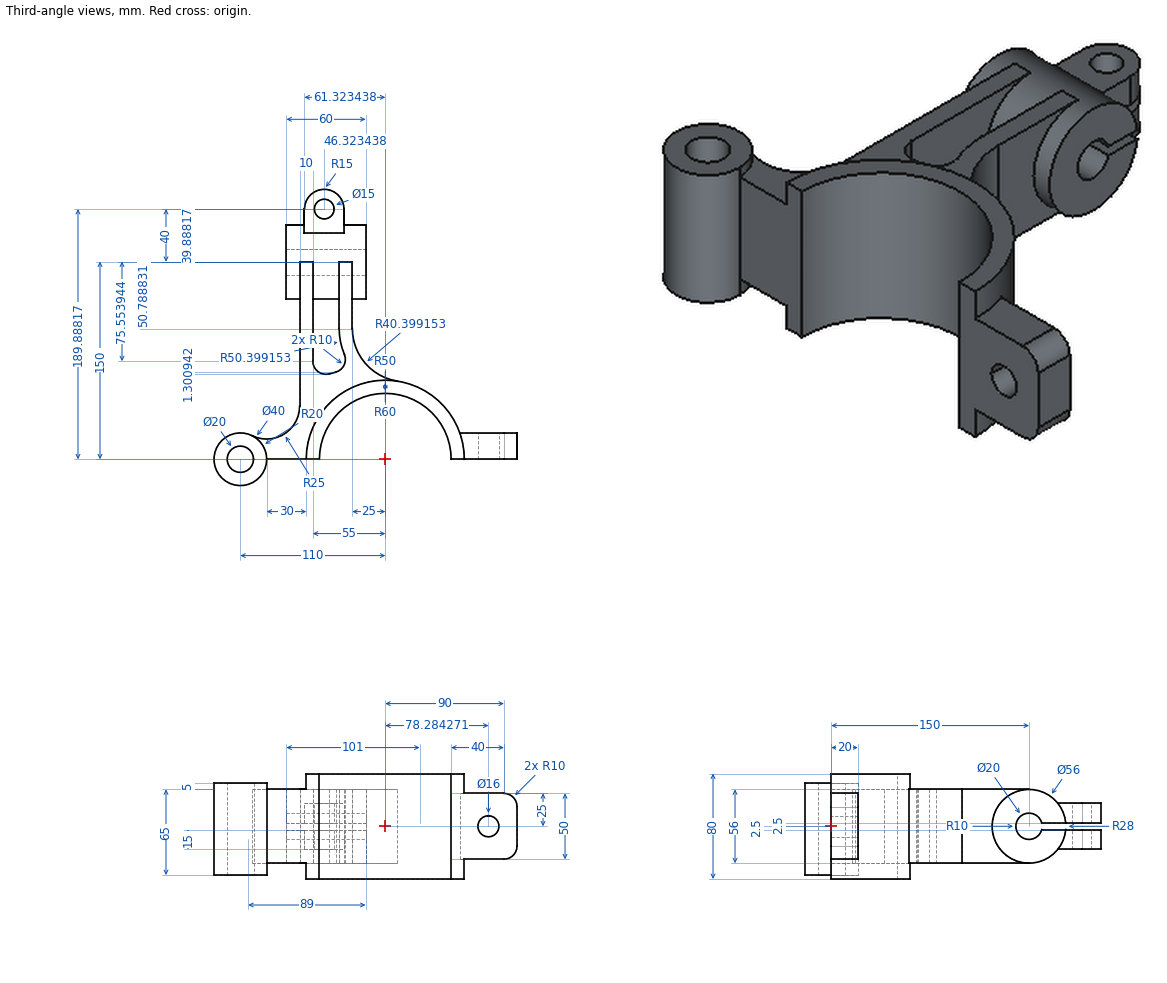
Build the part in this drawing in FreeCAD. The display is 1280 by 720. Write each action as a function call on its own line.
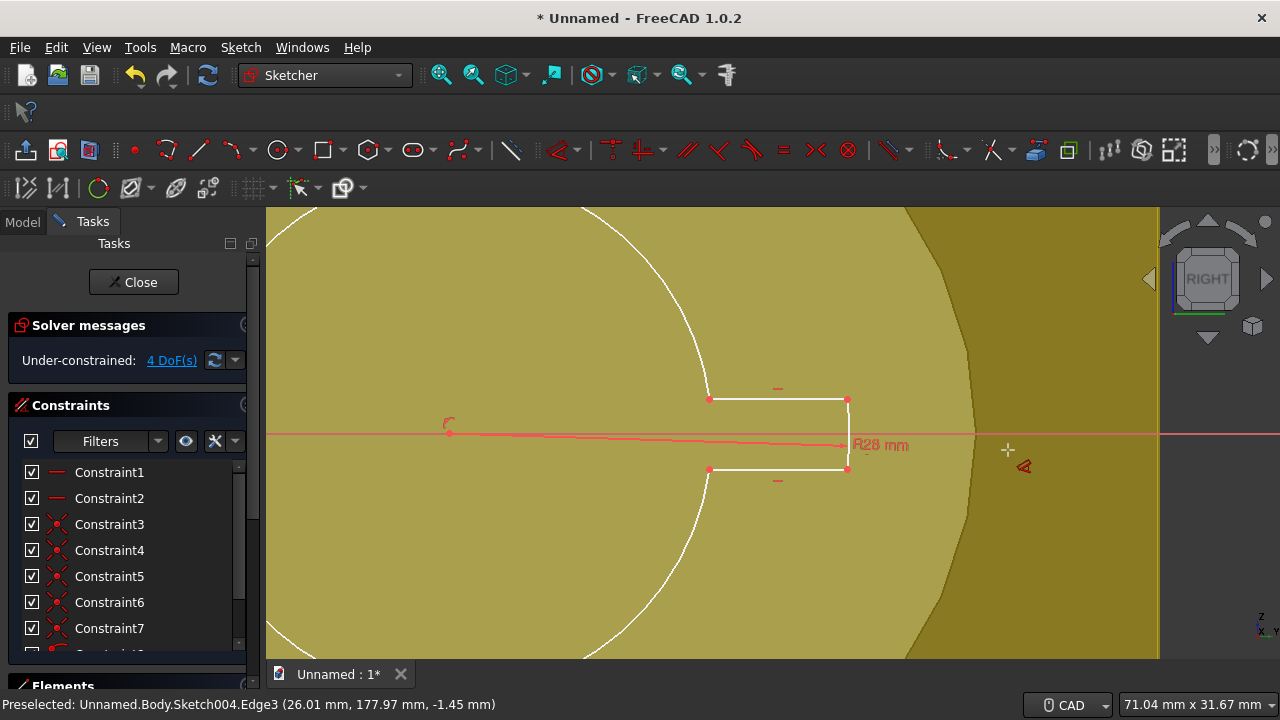
scroll(878, 631, down, 1)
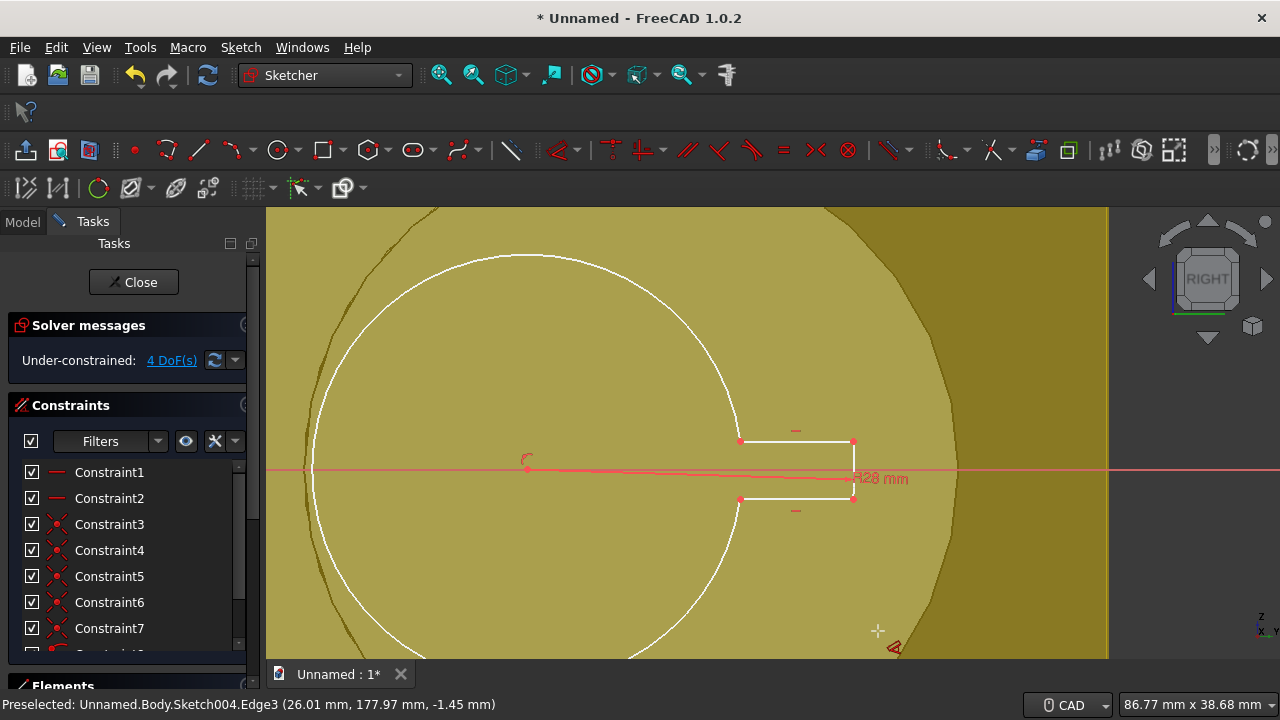
click(451, 269)
click(440, 239)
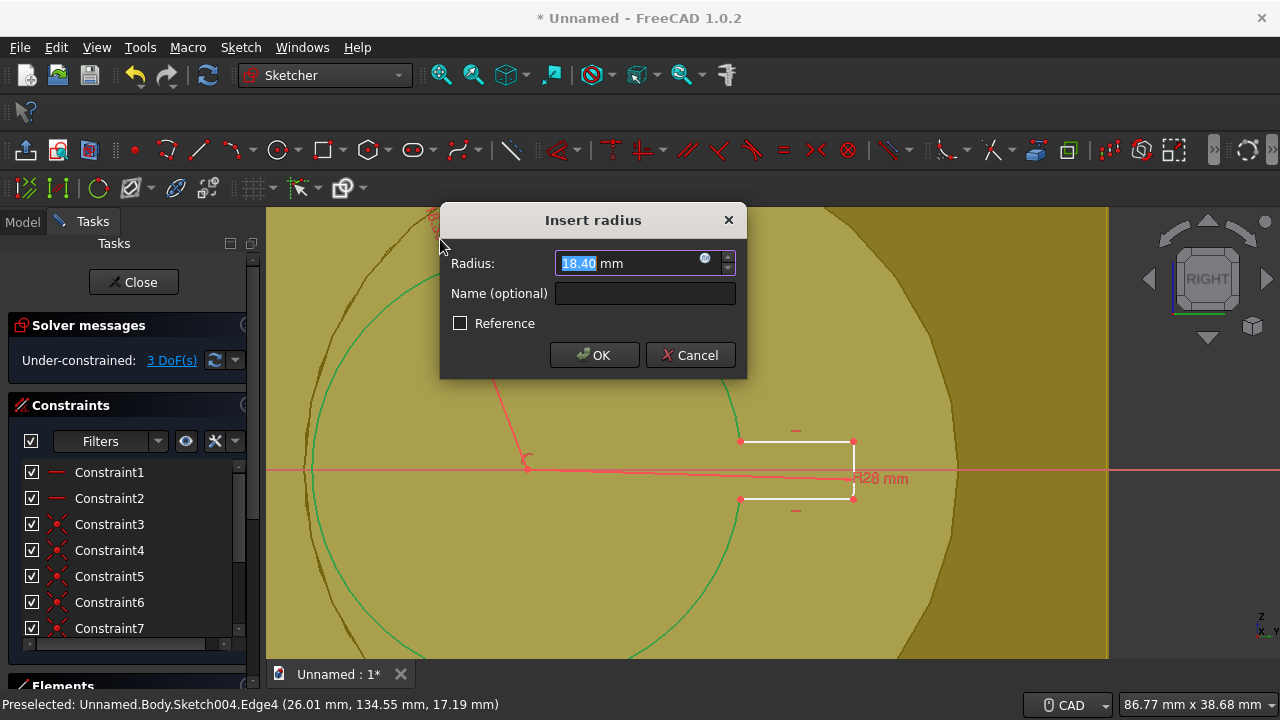
text(10)
key(Return)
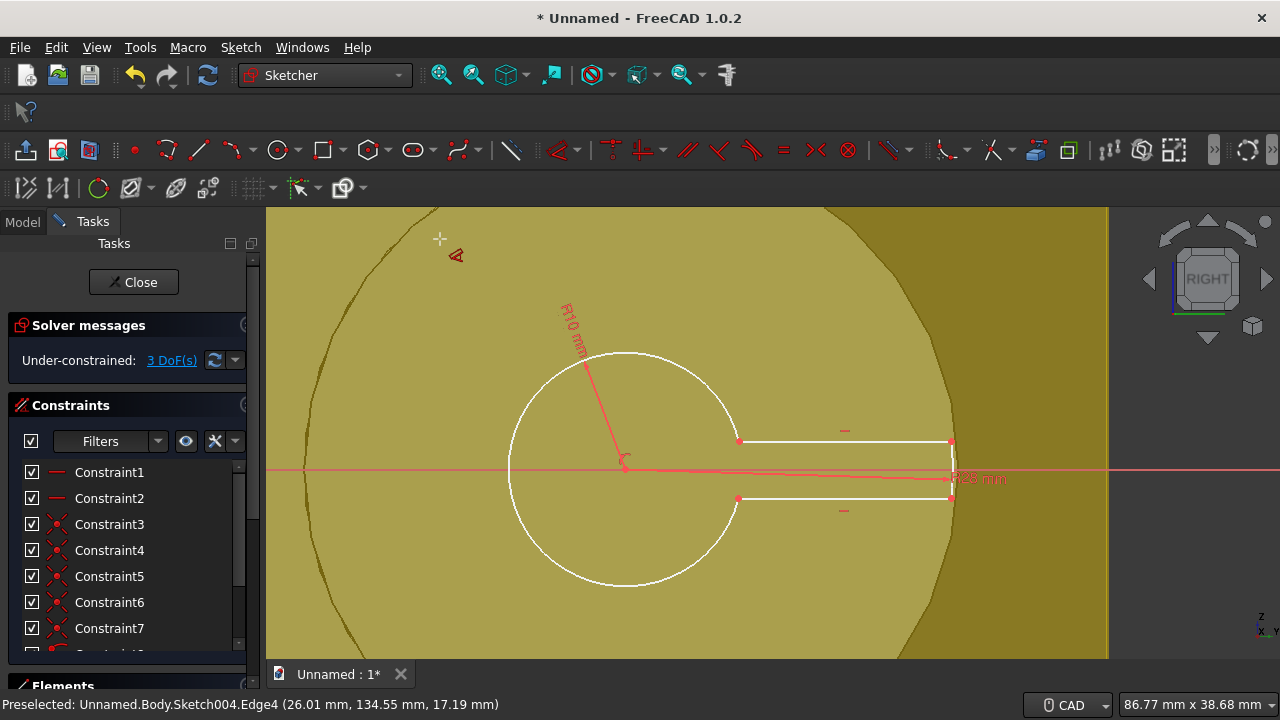
scroll(739, 442, up, 2)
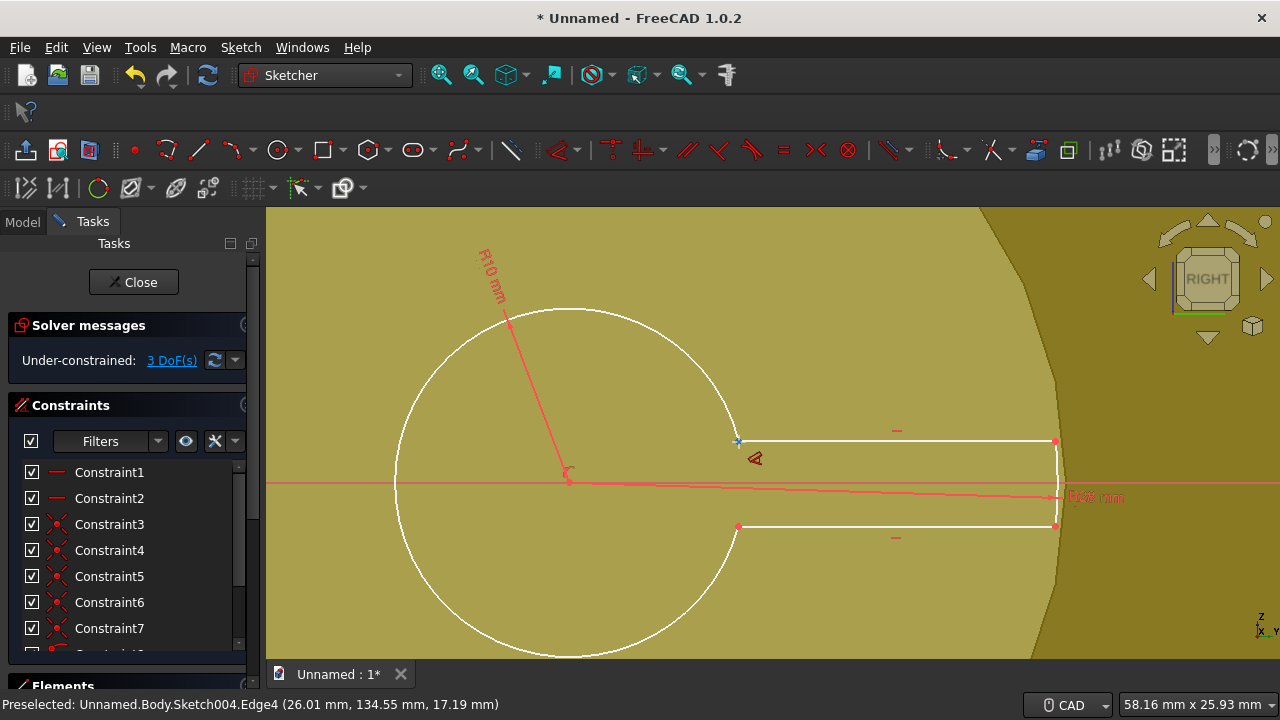
click(739, 441)
click(773, 462)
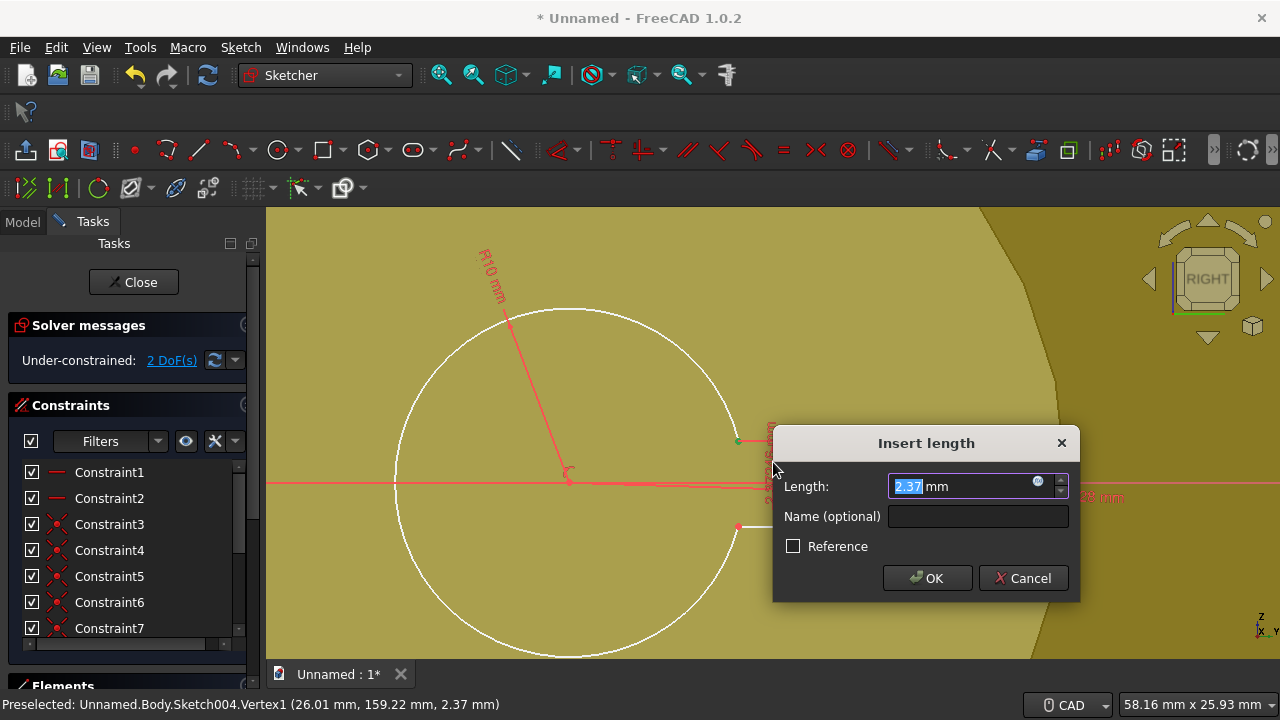
text(2.5)
key(Return)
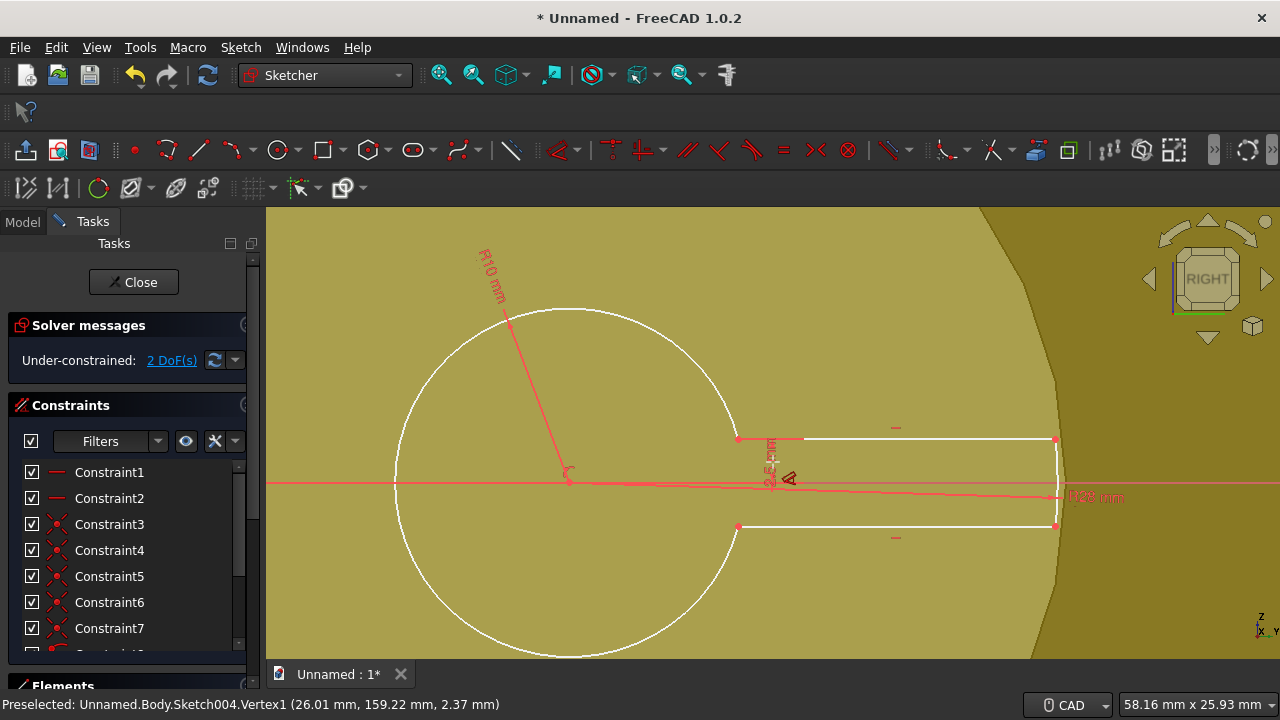
click(1056, 527)
click(1090, 515)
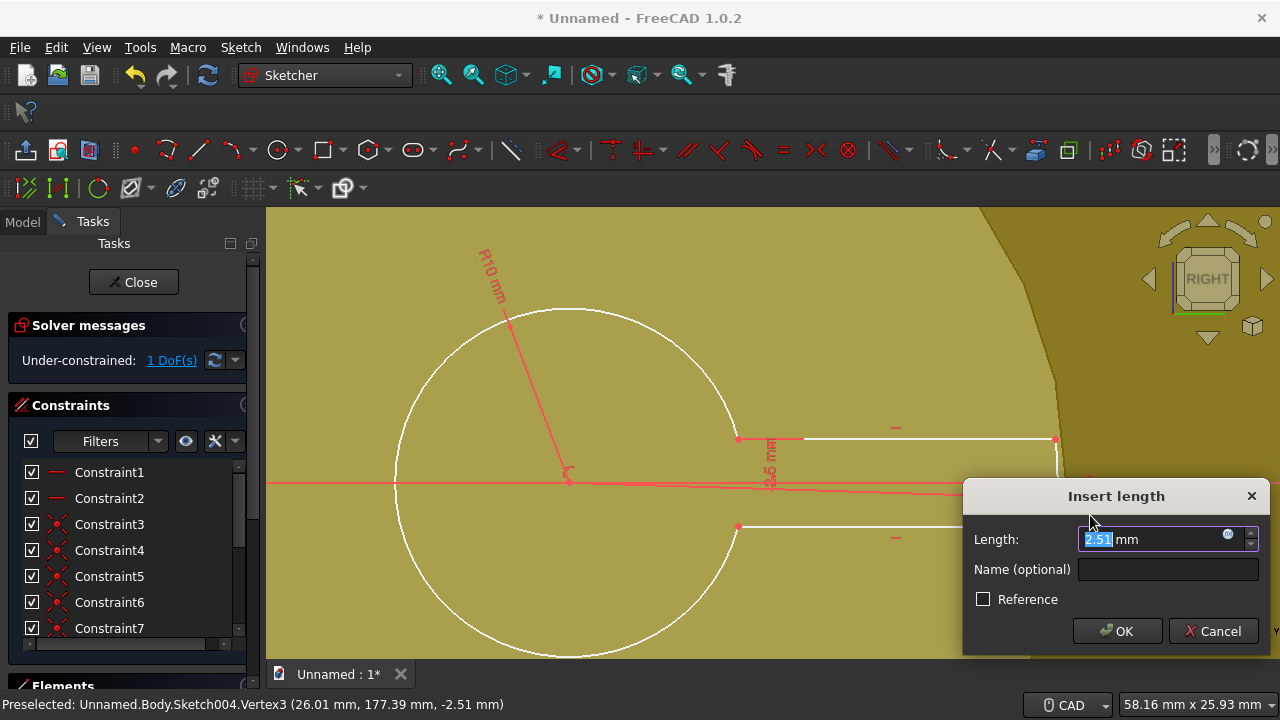
text(2.5)
key(Return)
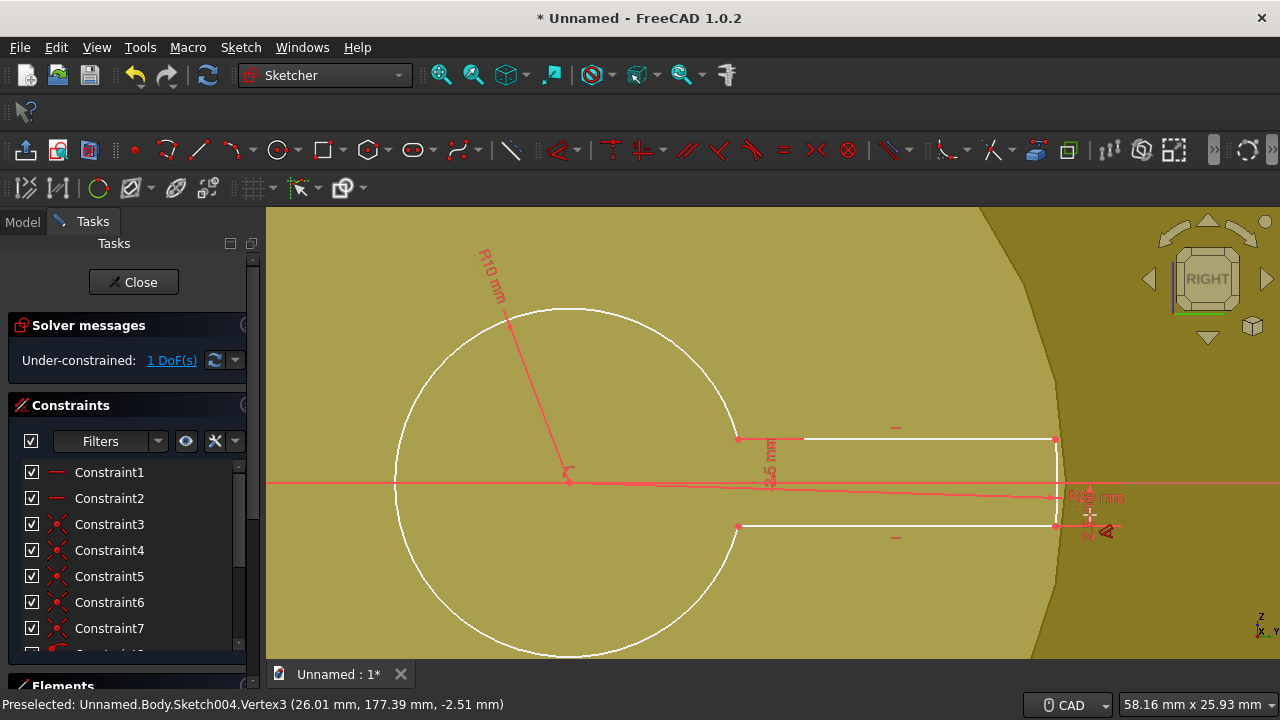
click(569, 483)
click(432, 517)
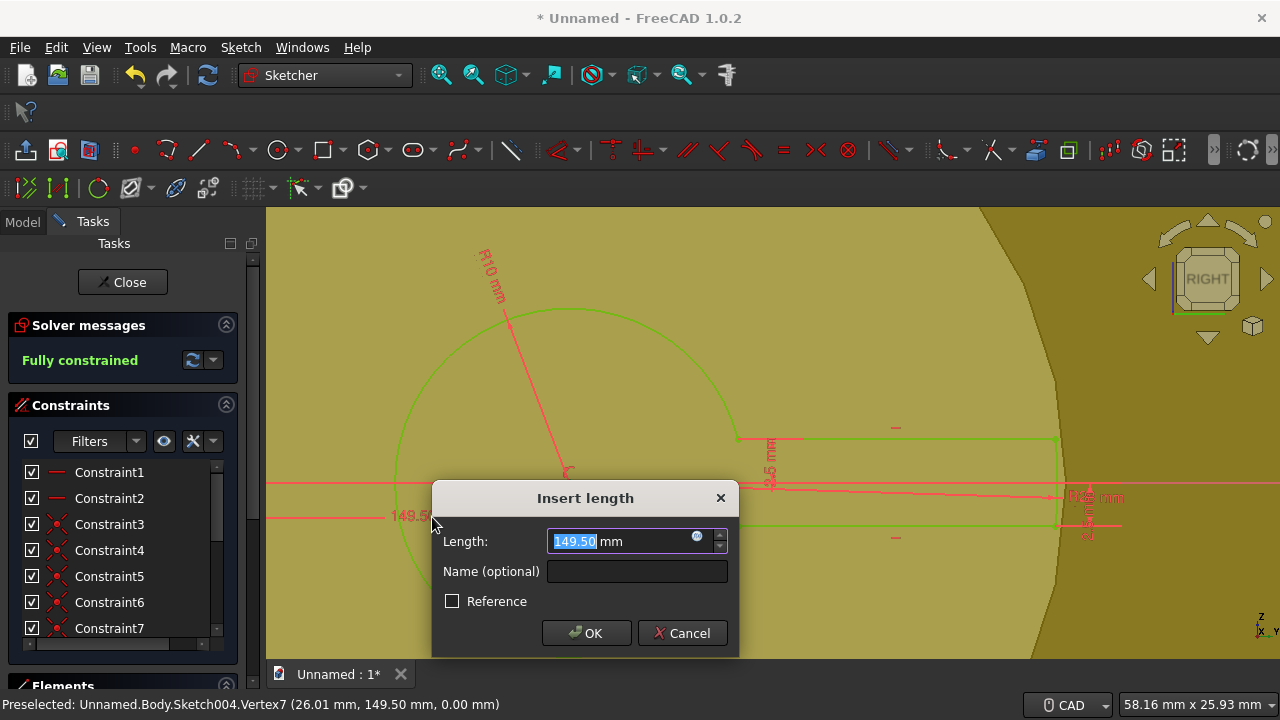
text(150)
key(Return)
key(Escape)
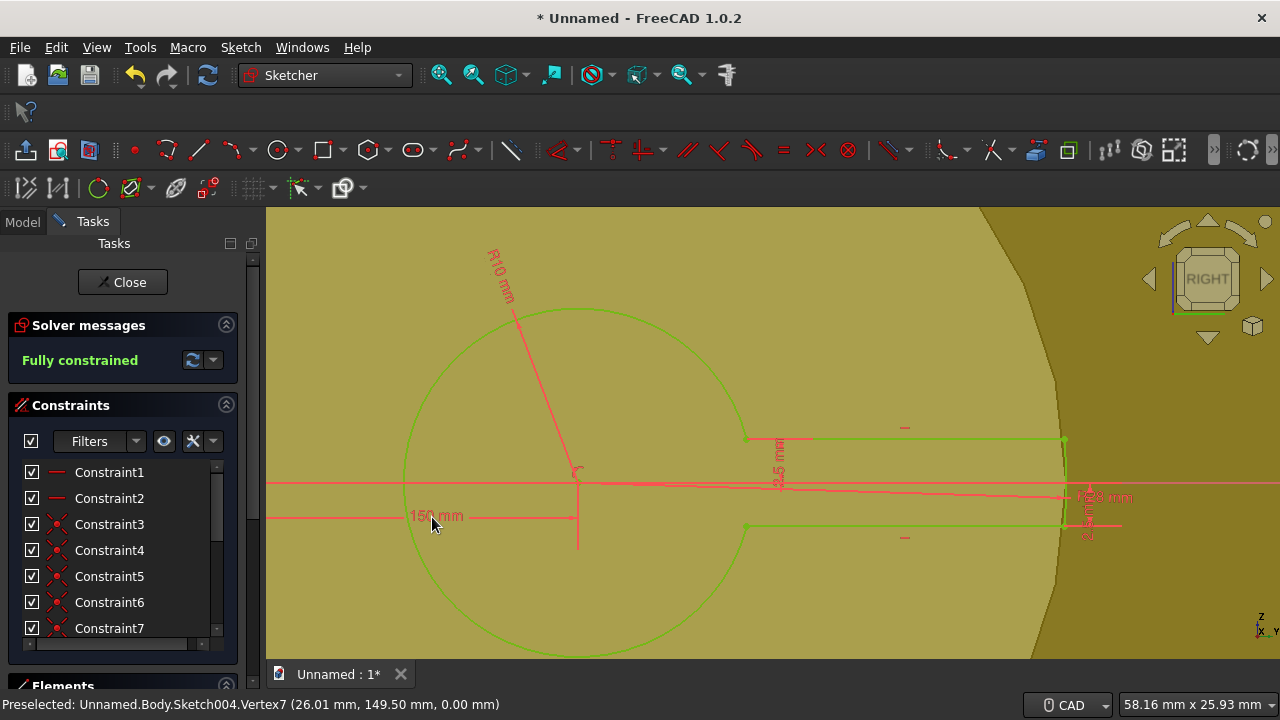
click(123, 282)